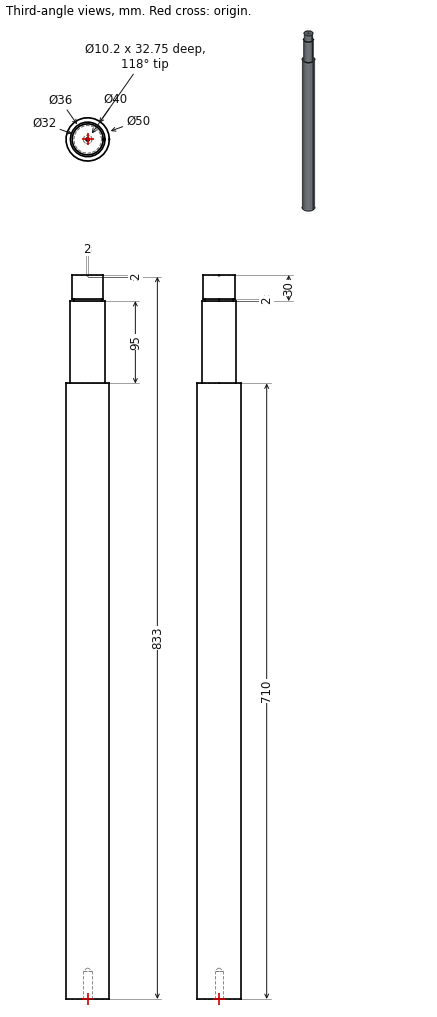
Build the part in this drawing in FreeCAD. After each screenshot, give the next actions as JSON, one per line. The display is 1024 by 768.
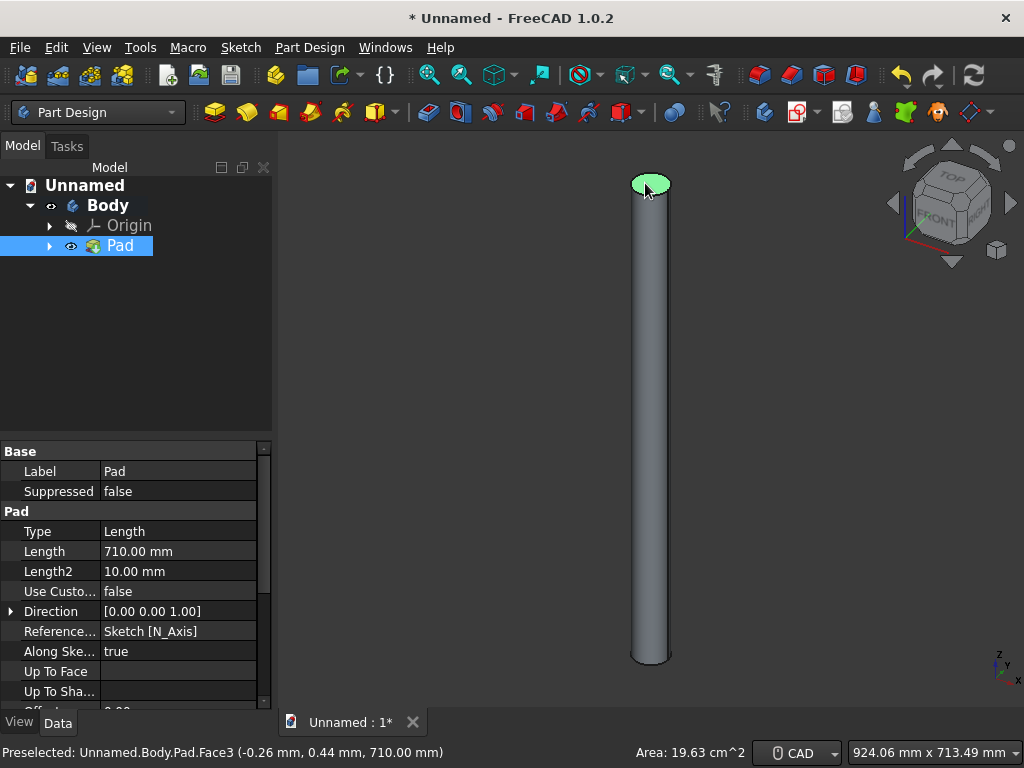
{"action": "left_click", "coordinate": [798, 112]}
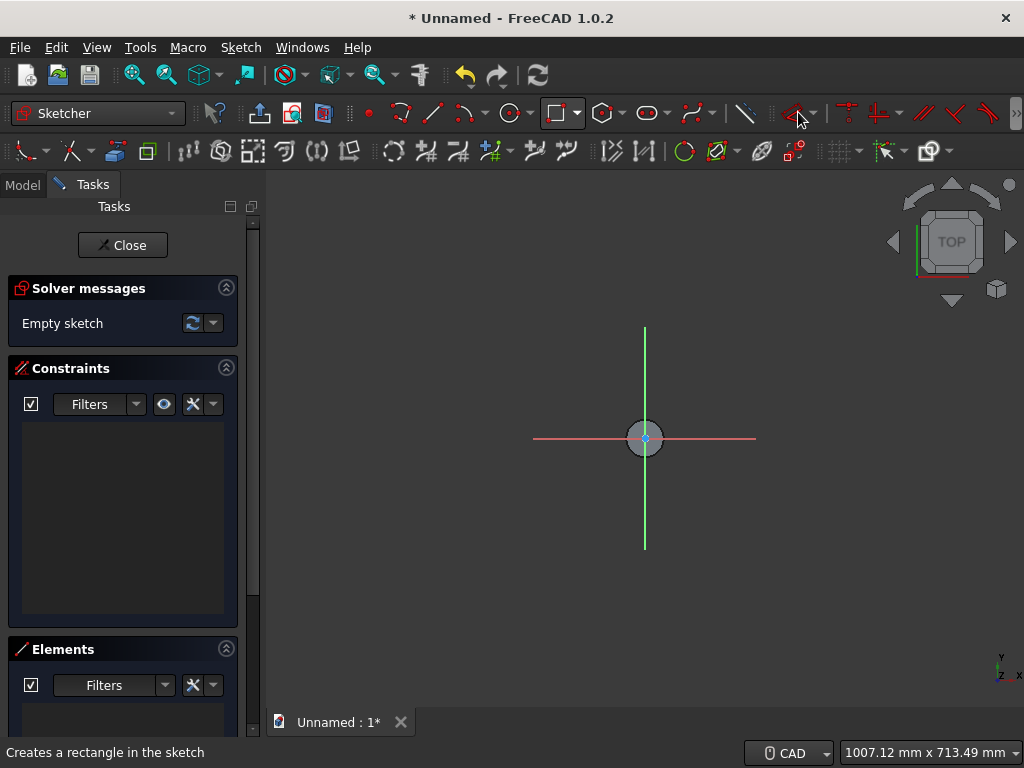
{"action": "scroll", "coordinate": [652, 438], "scroll_direction": "up", "scroll_amount": 12}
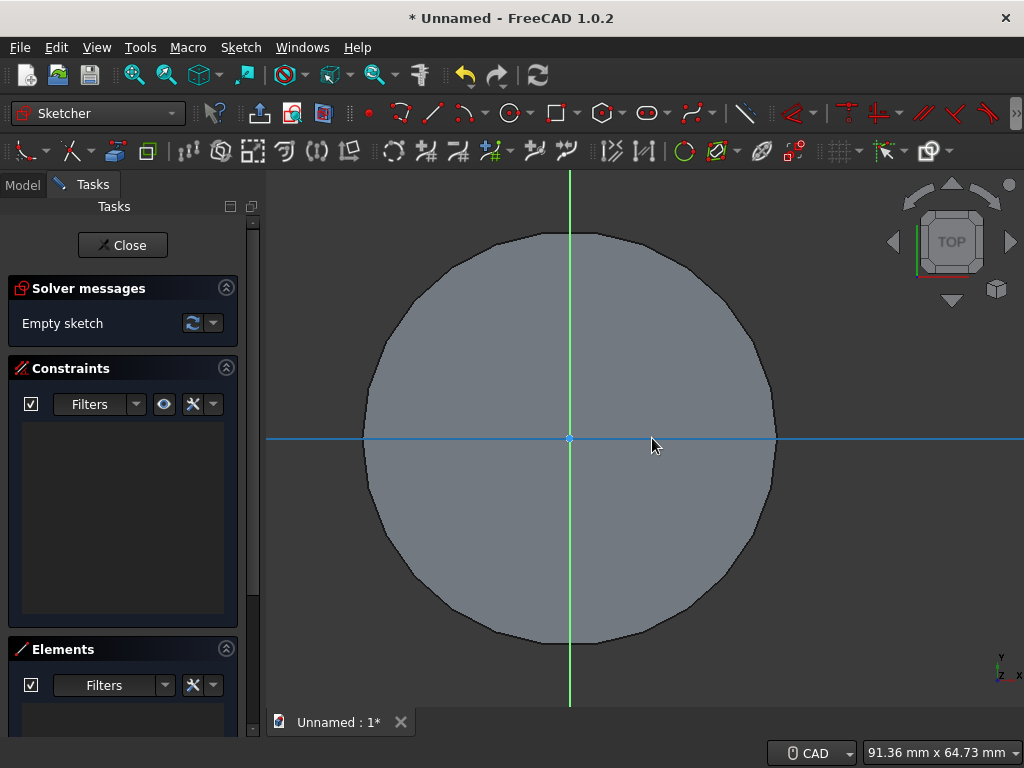
{"action": "left_click", "coordinate": [510, 114]}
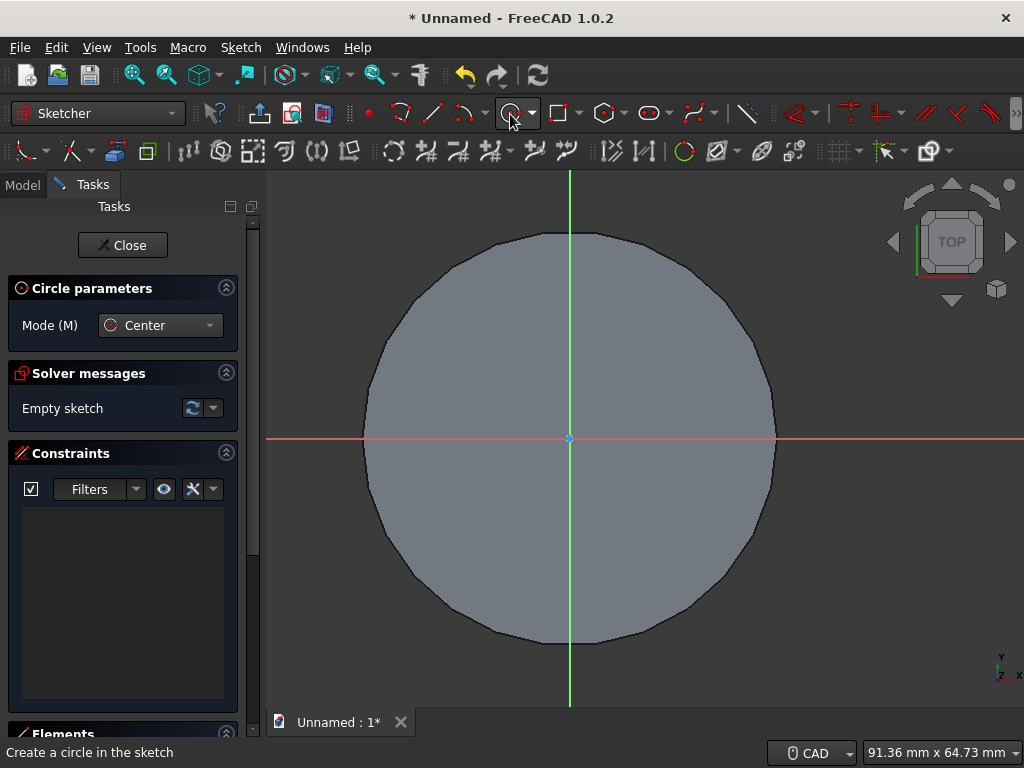
{"action": "left_click", "coordinate": [570, 438]}
{"action": "mouse_move", "coordinate": [687, 321]}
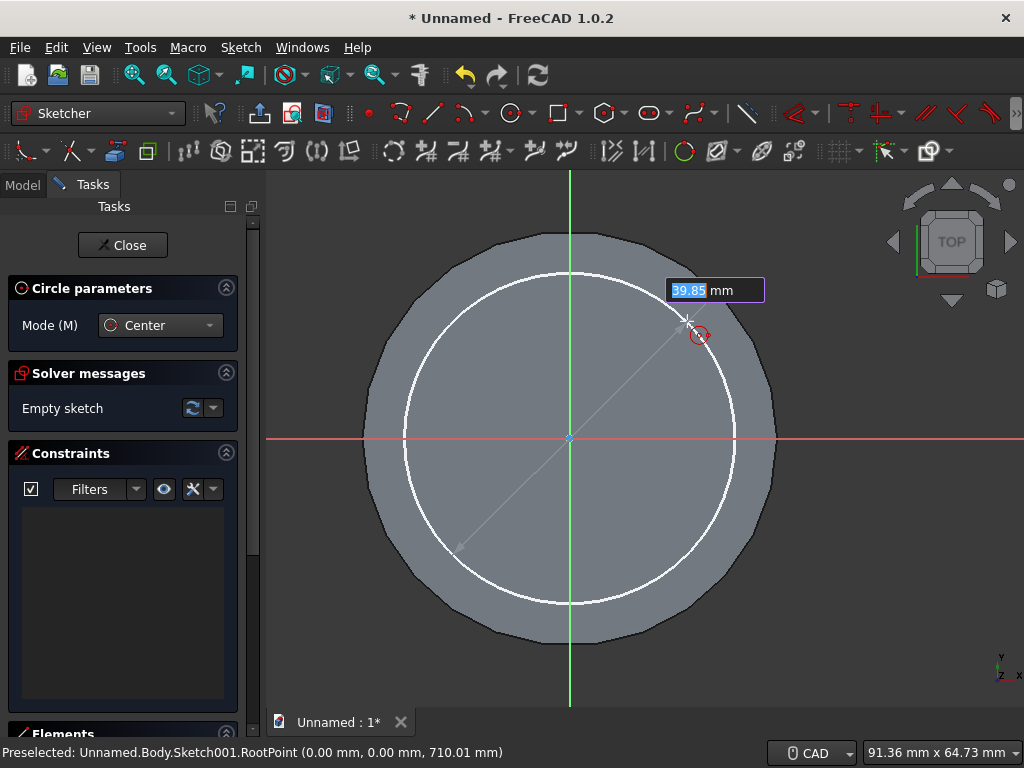
{"action": "type", "text": "40"}
{"action": "key", "text": "Return"}
{"action": "key", "text": "Escape"}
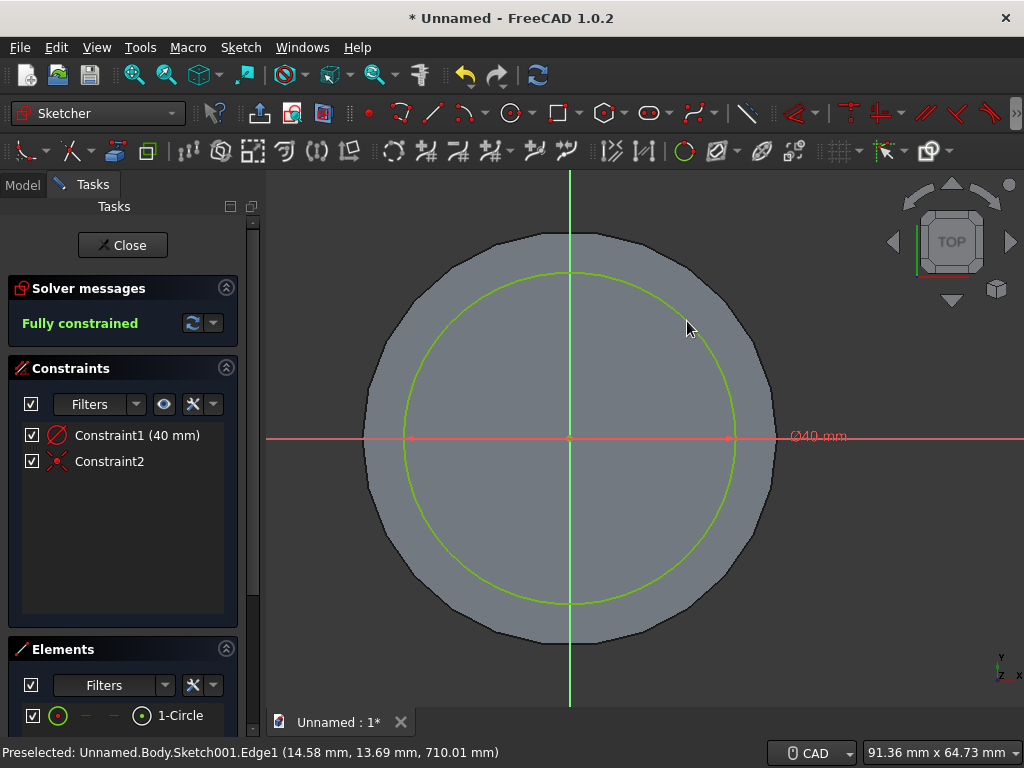
{"action": "left_click", "coordinate": [123, 245]}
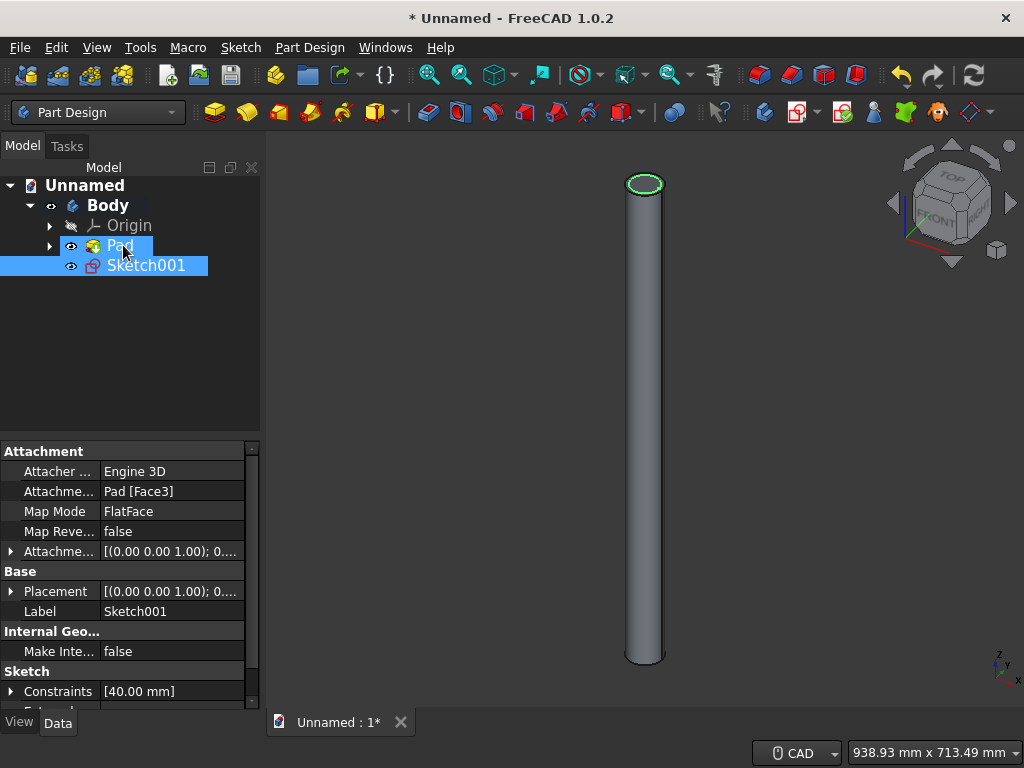
{"action": "left_click", "coordinate": [216, 112]}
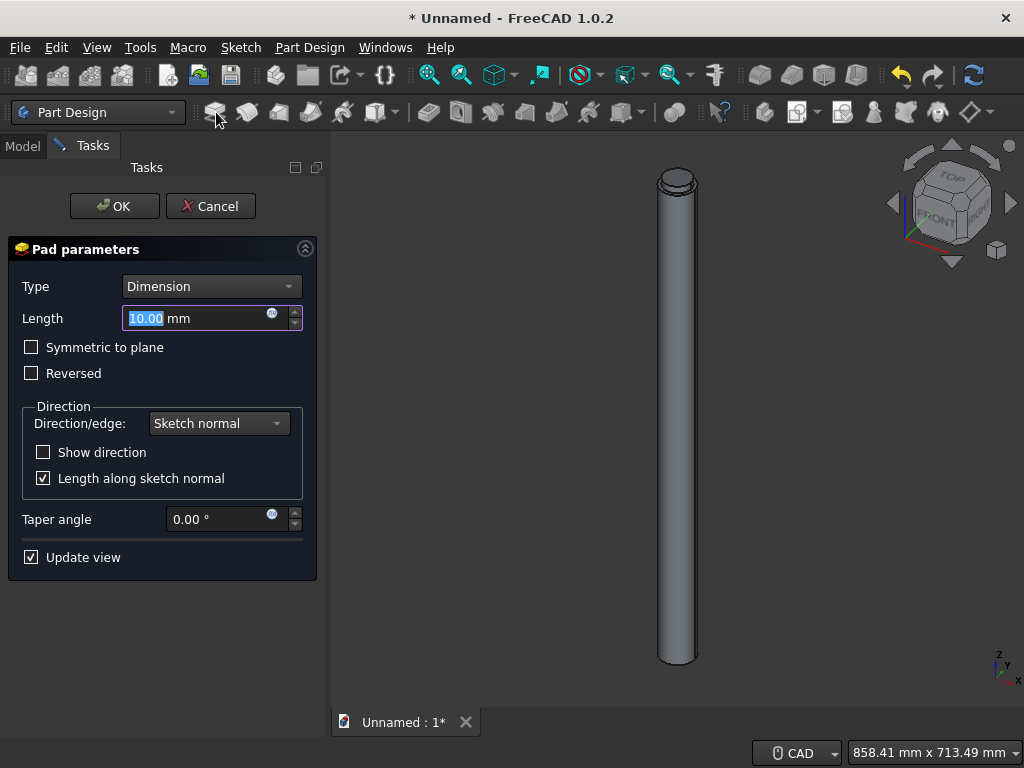
{"action": "type", "text": "95"}
{"action": "key", "text": "Tab"}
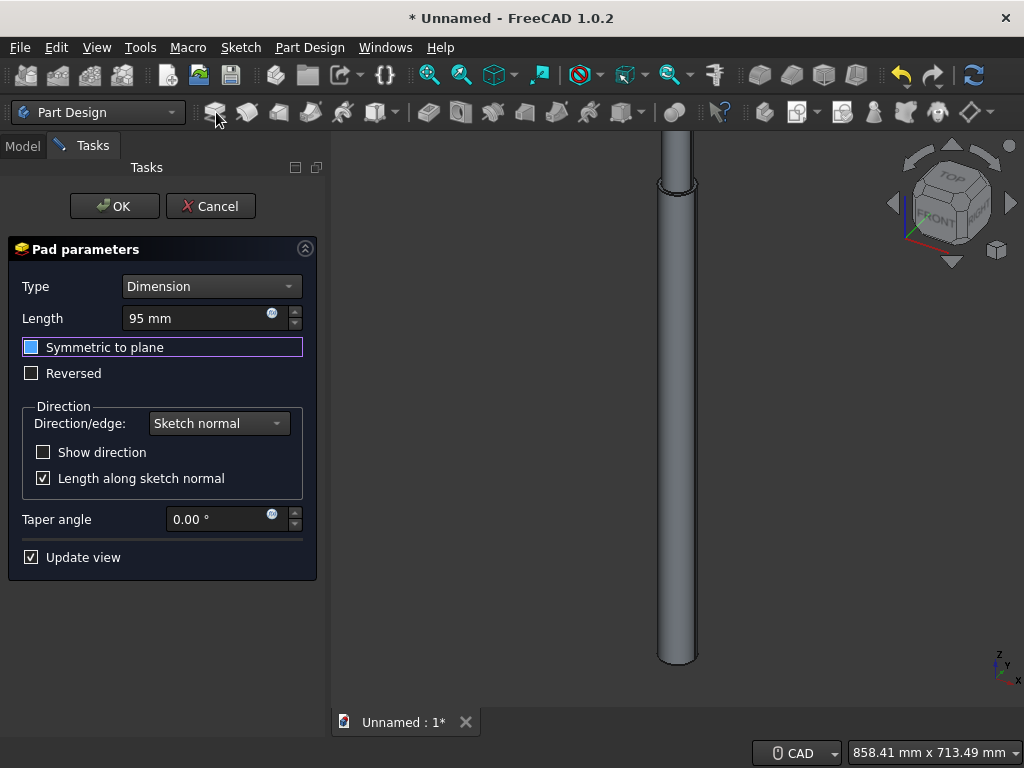
{"action": "left_click", "coordinate": [115, 206]}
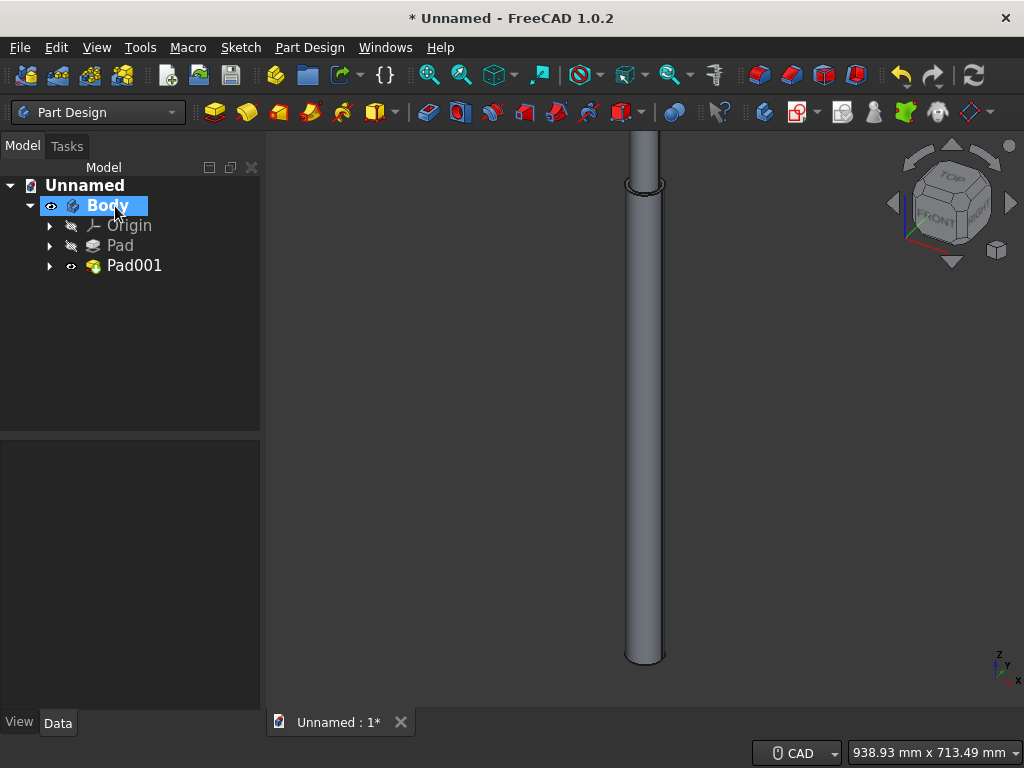
{"action": "left_click", "coordinate": [430, 76]}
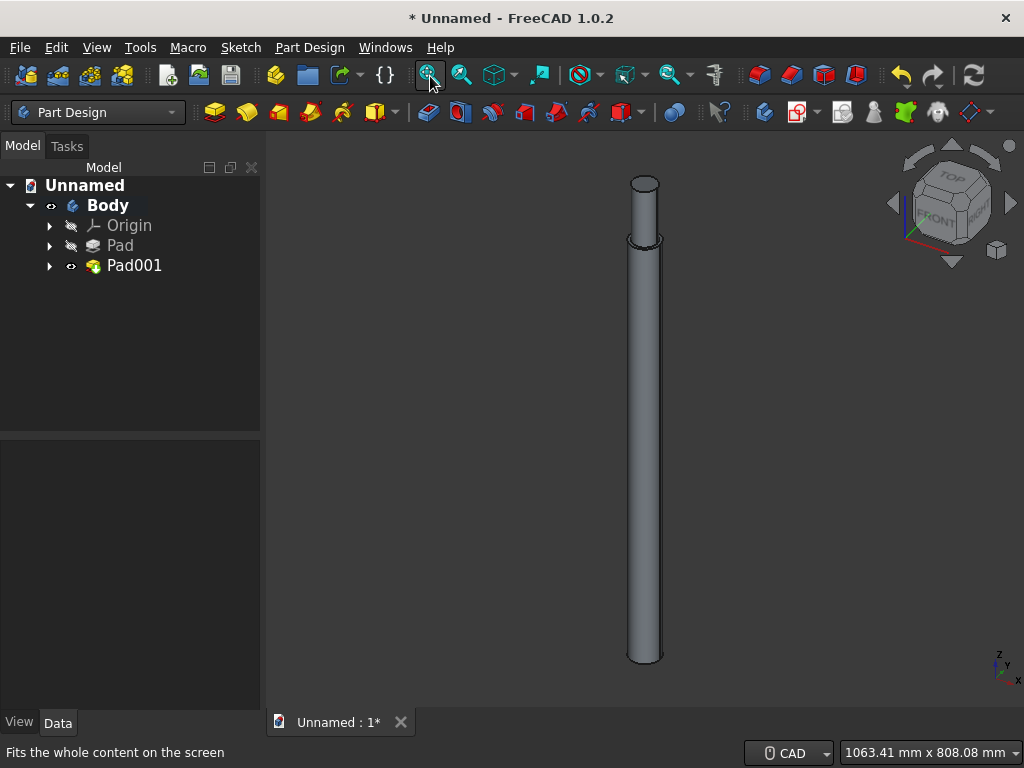
{"action": "left_click", "coordinate": [647, 181]}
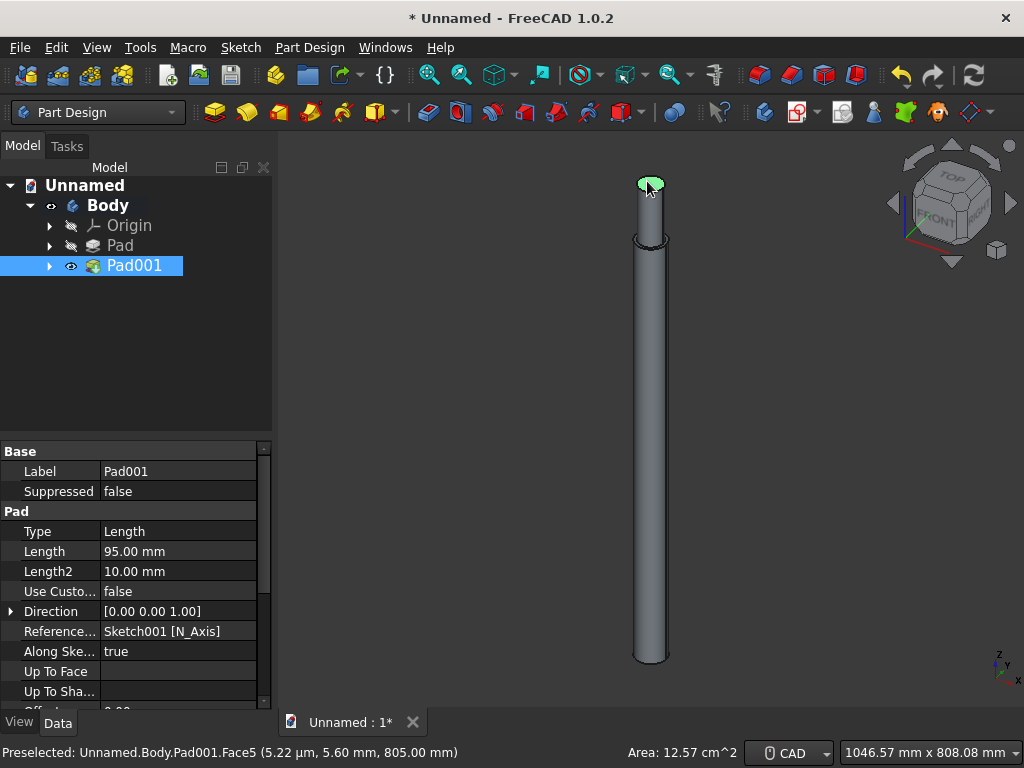
{"action": "left_click", "coordinate": [798, 112]}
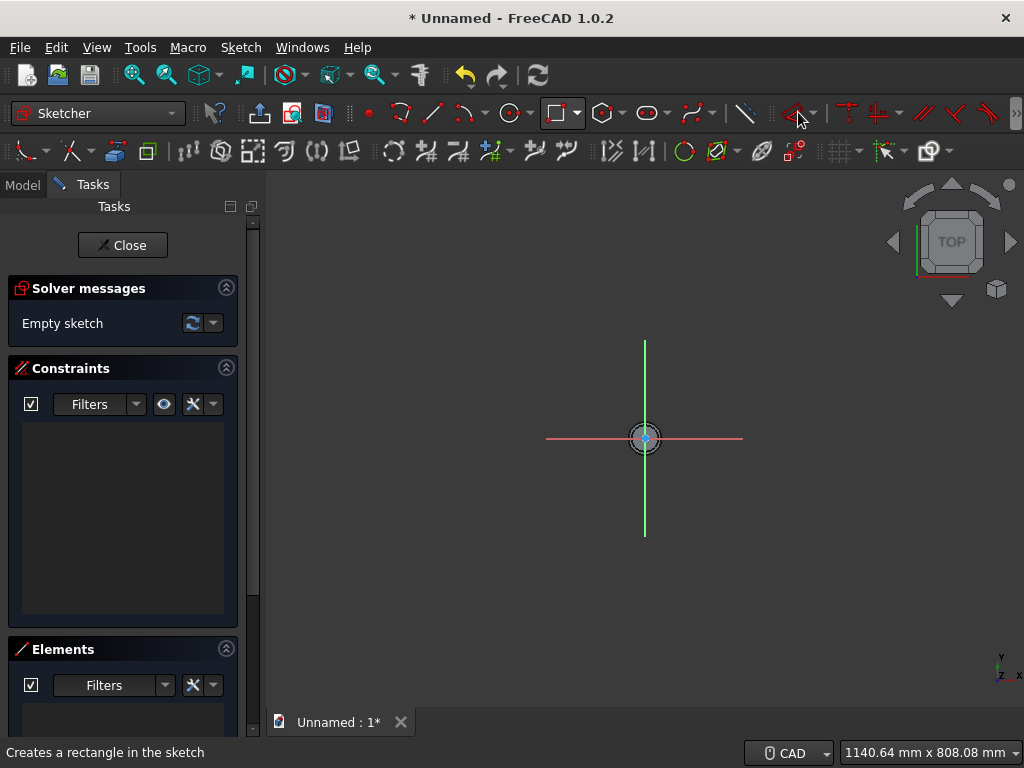
{"action": "scroll", "coordinate": [650, 438], "scroll_direction": "up", "scroll_amount": 13}